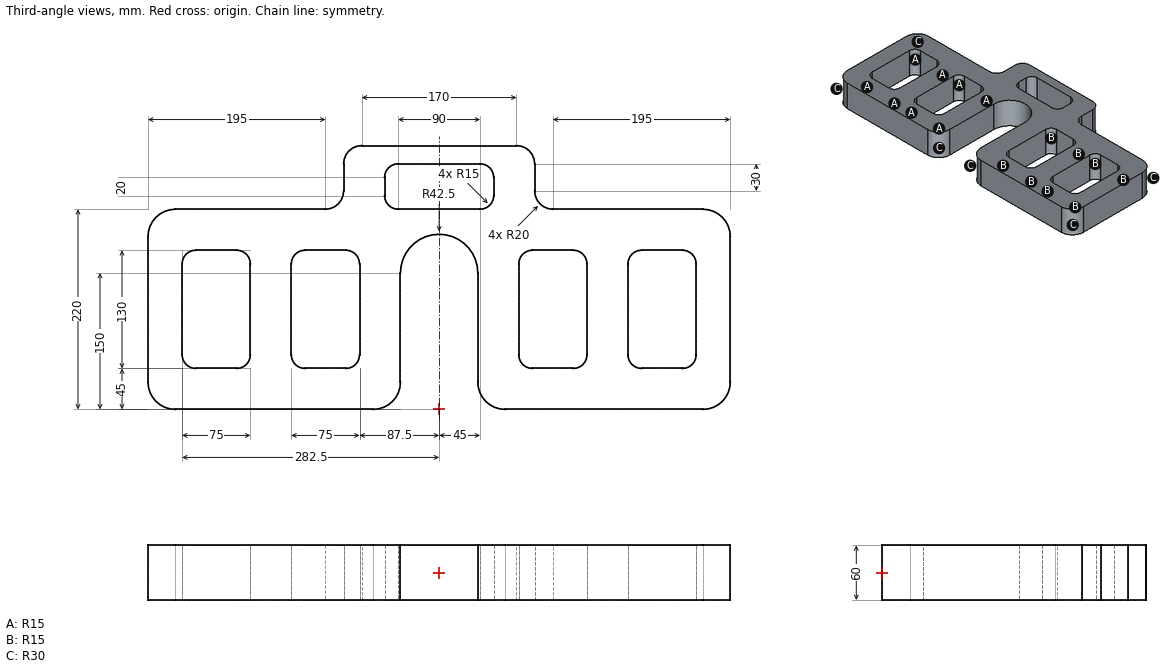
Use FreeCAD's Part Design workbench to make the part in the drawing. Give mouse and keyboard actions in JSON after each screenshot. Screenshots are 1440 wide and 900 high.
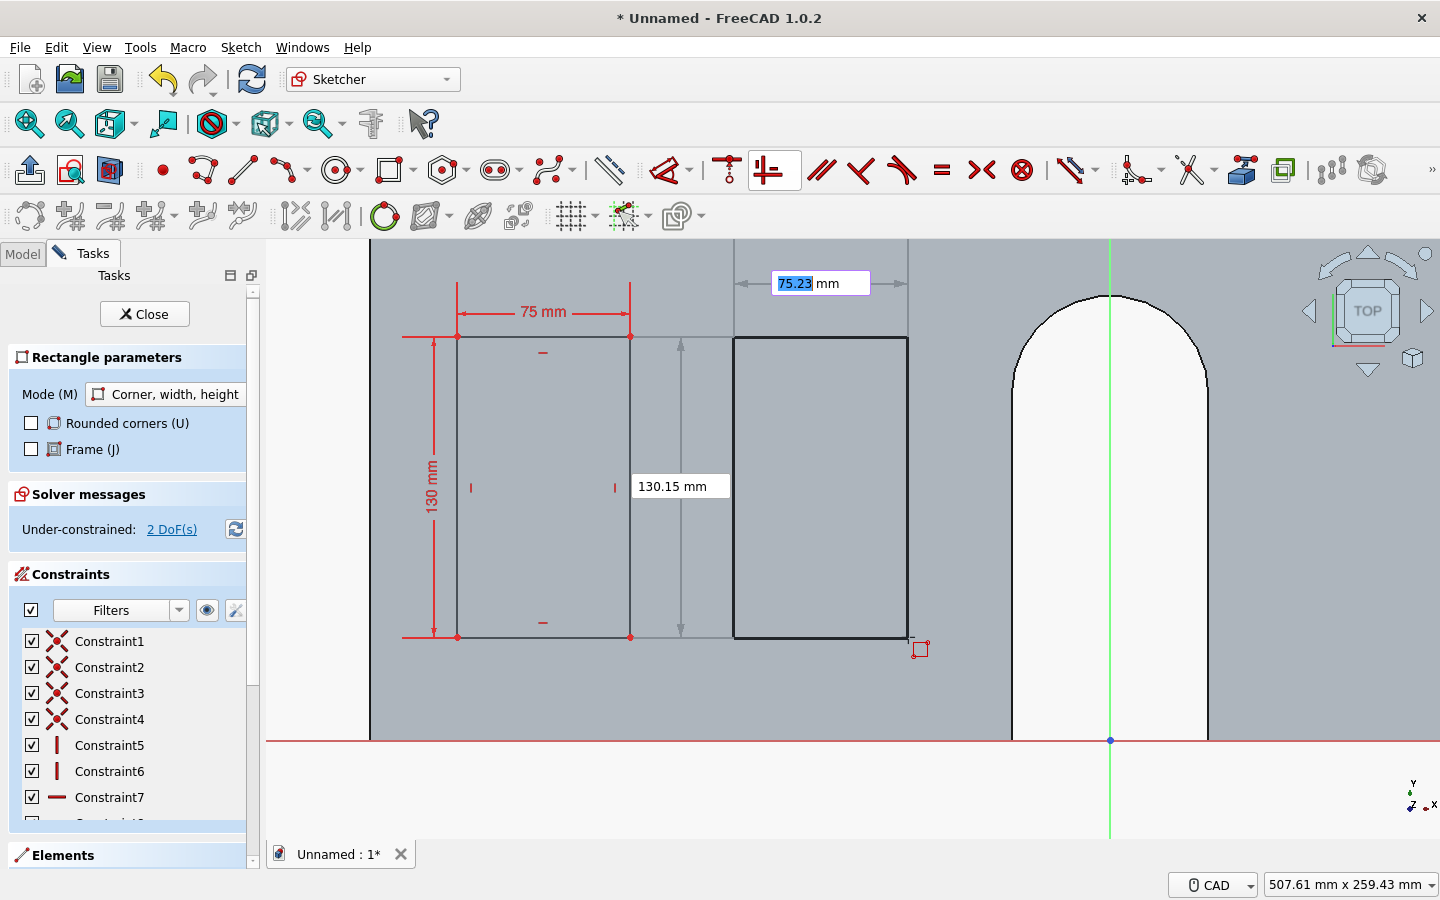
{"action": "type", "text": "75"}
{"action": "key", "text": "Tab"}
{"action": "type", "text": "130"}
{"action": "key", "text": "Return"}
{"action": "key", "text": "Escape"}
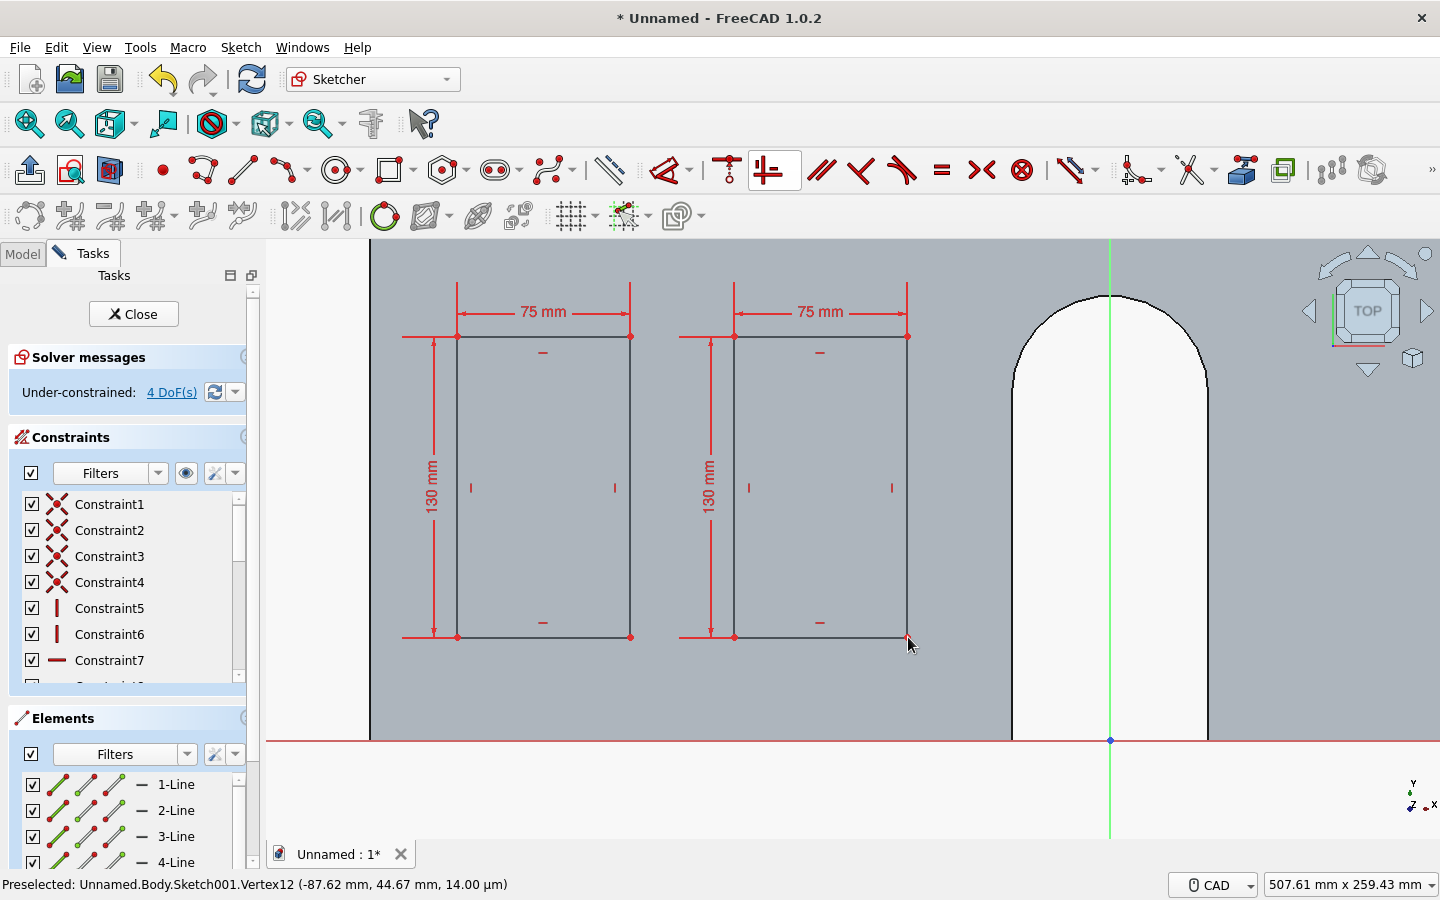
{"action": "left_click", "coordinate": [664, 170]}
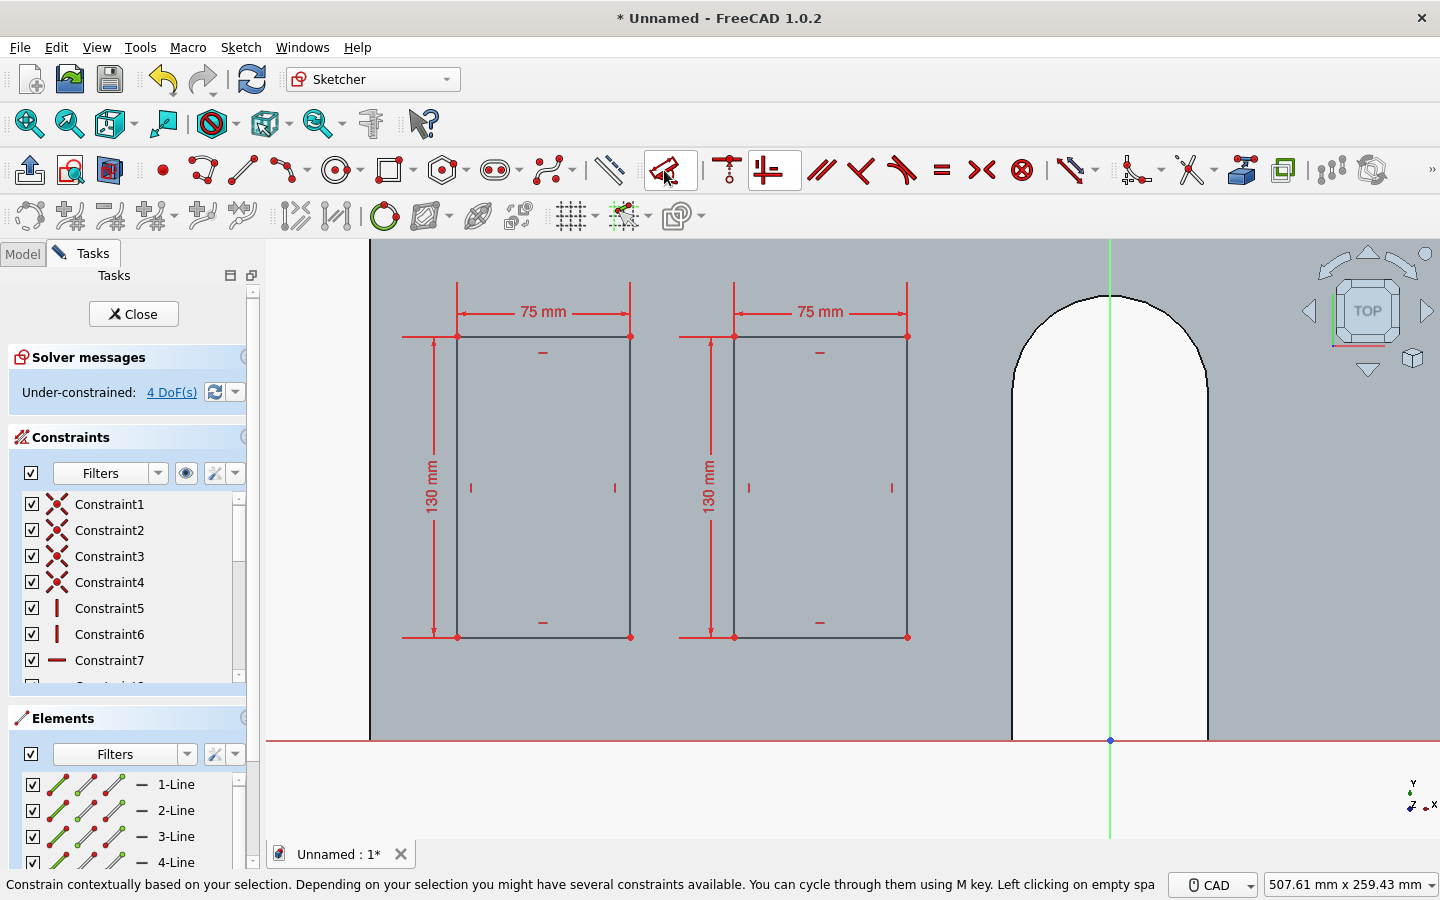
{"action": "left_click", "coordinate": [457, 638]}
{"action": "left_click", "coordinate": [1144, 689]}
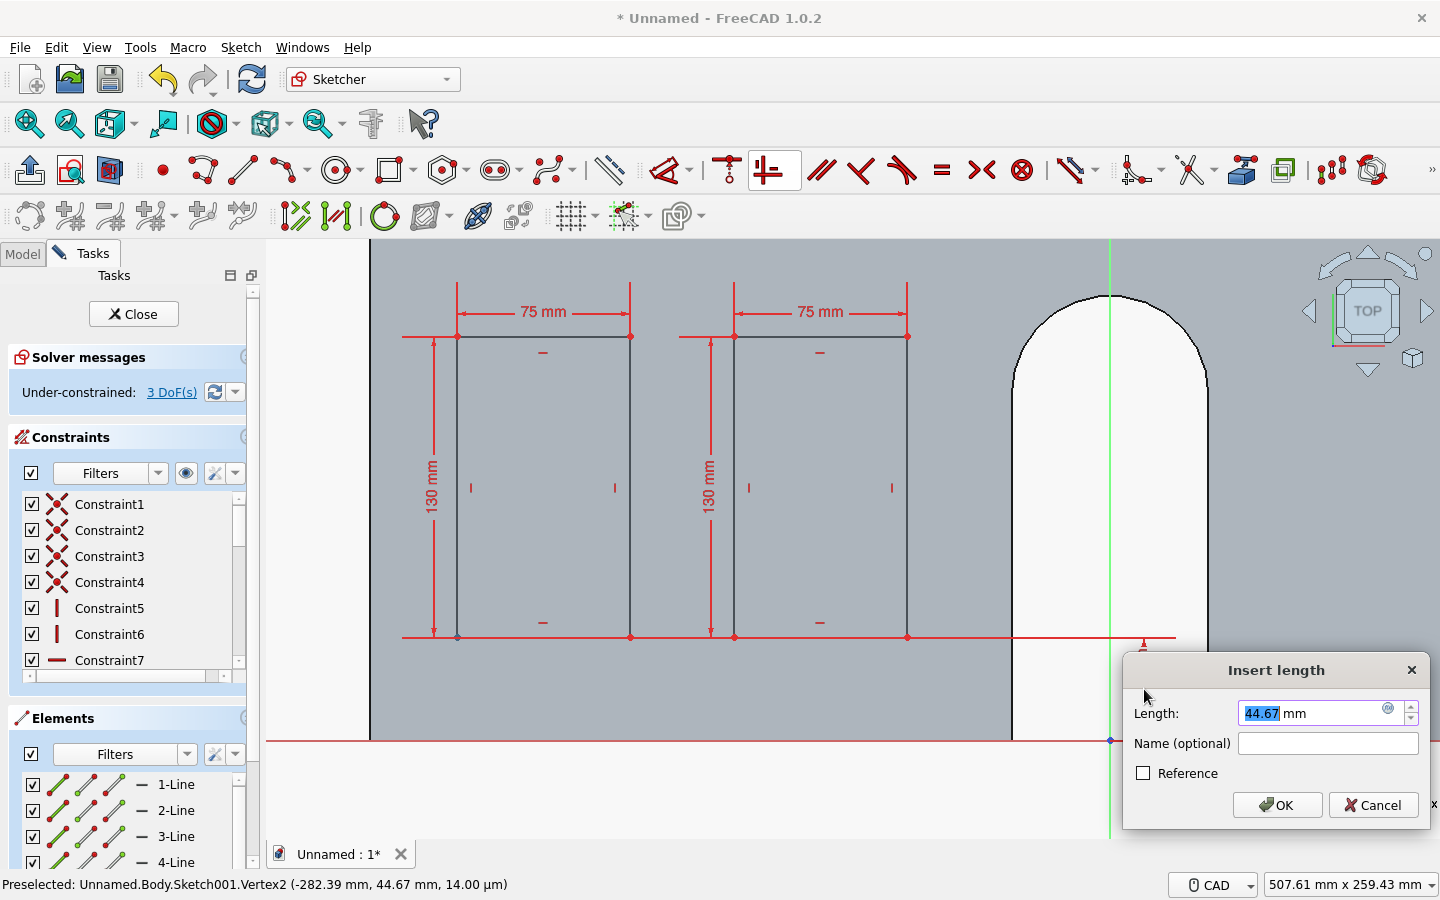
{"action": "type", "text": "45"}
{"action": "key", "text": "Return"}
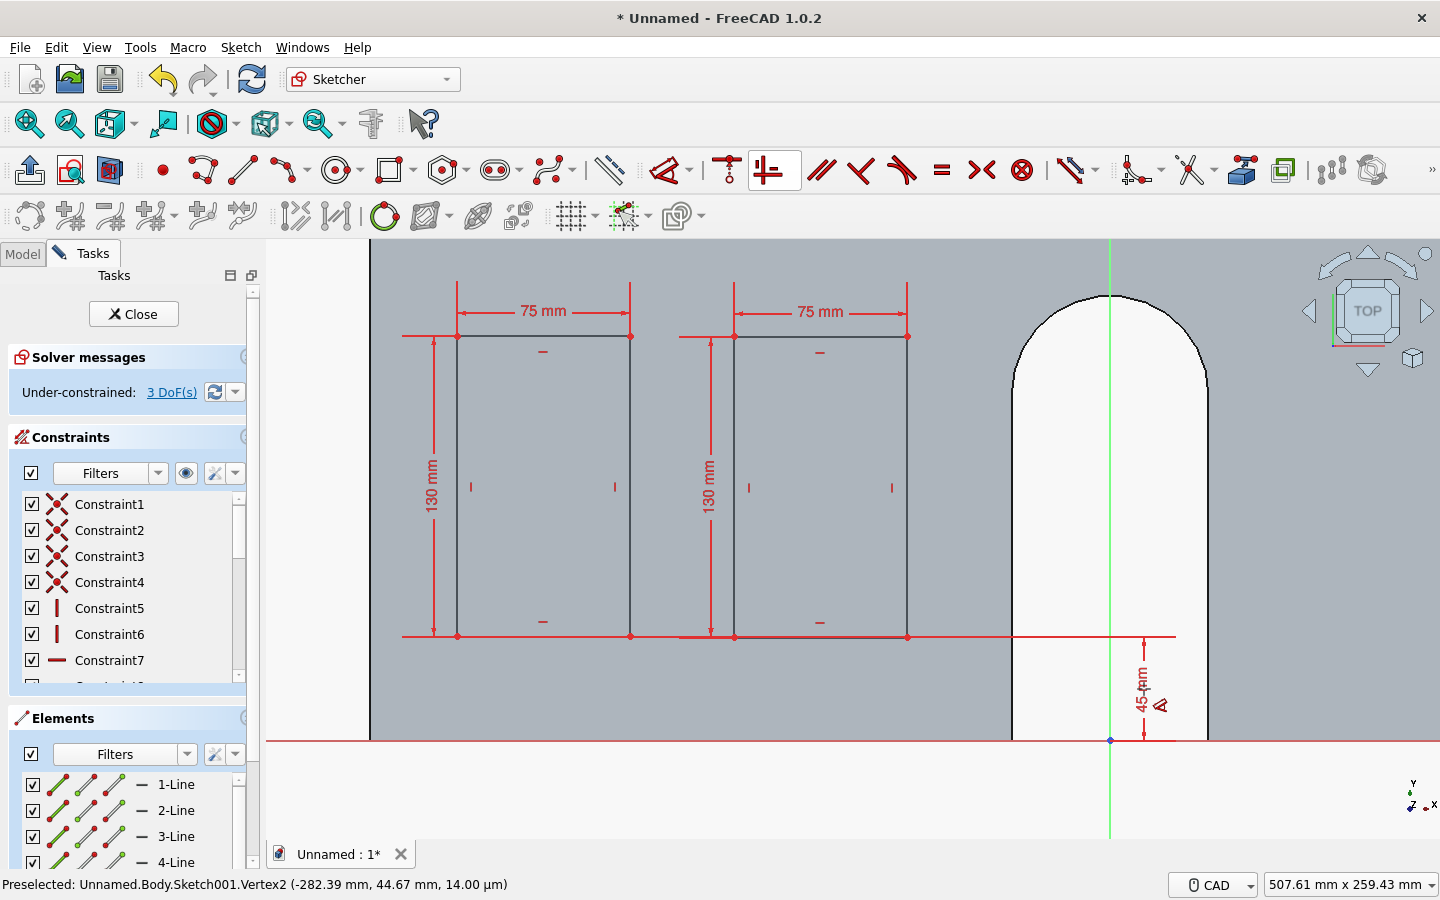
{"action": "left_click", "coordinate": [734, 638]}
{"action": "left_click", "coordinate": [1144, 666]}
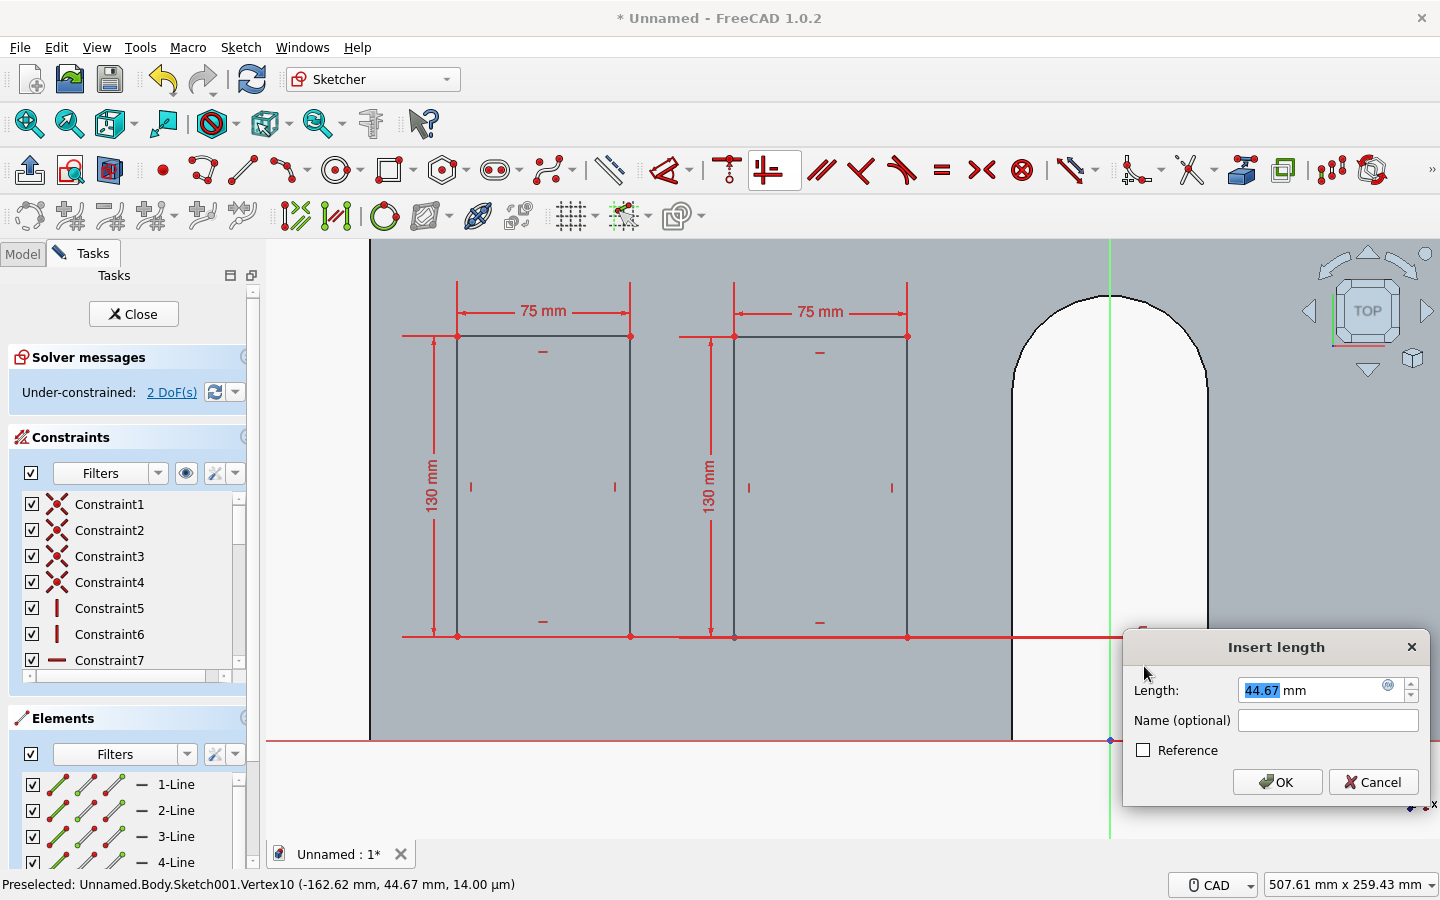
{"action": "type", "text": "45"}
{"action": "key", "text": "Return"}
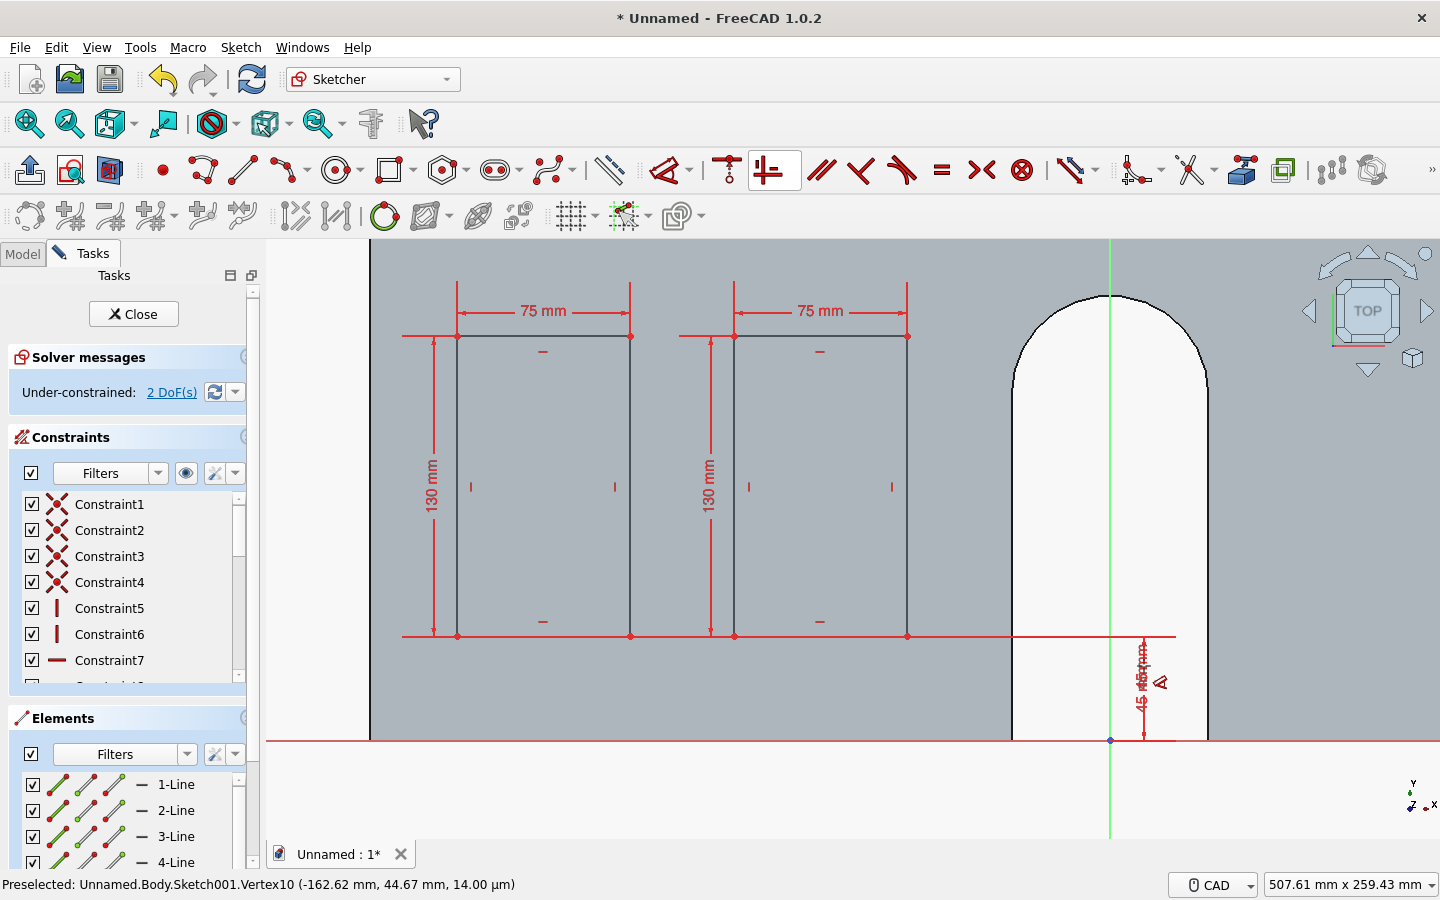
{"action": "left_click", "coordinate": [907, 637]}
{"action": "left_click", "coordinate": [1009, 775]}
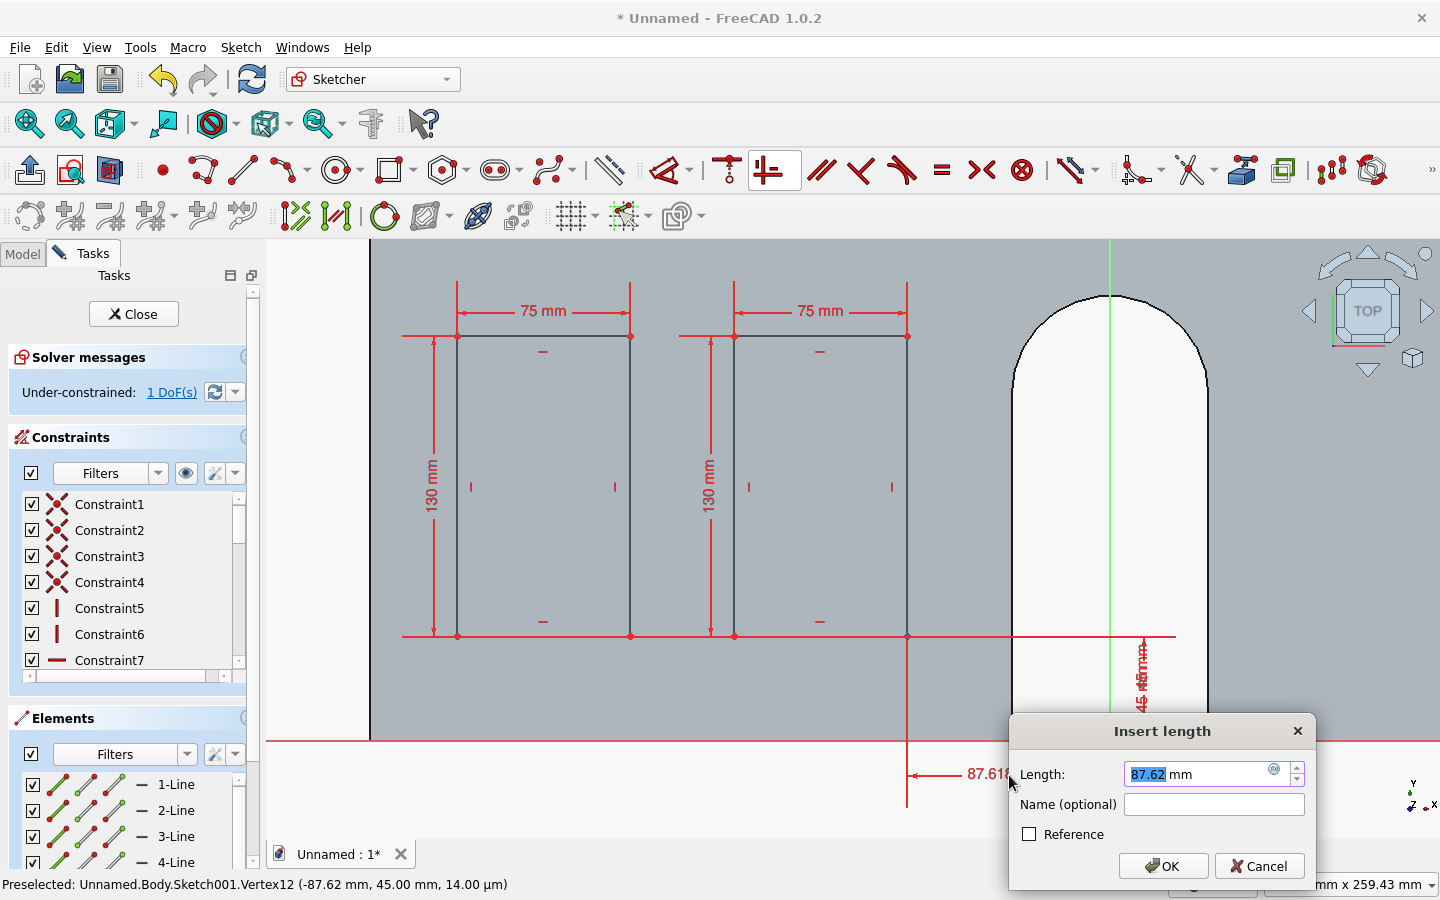
{"action": "type", "text": "87.5"}
{"action": "key", "text": "Return"}